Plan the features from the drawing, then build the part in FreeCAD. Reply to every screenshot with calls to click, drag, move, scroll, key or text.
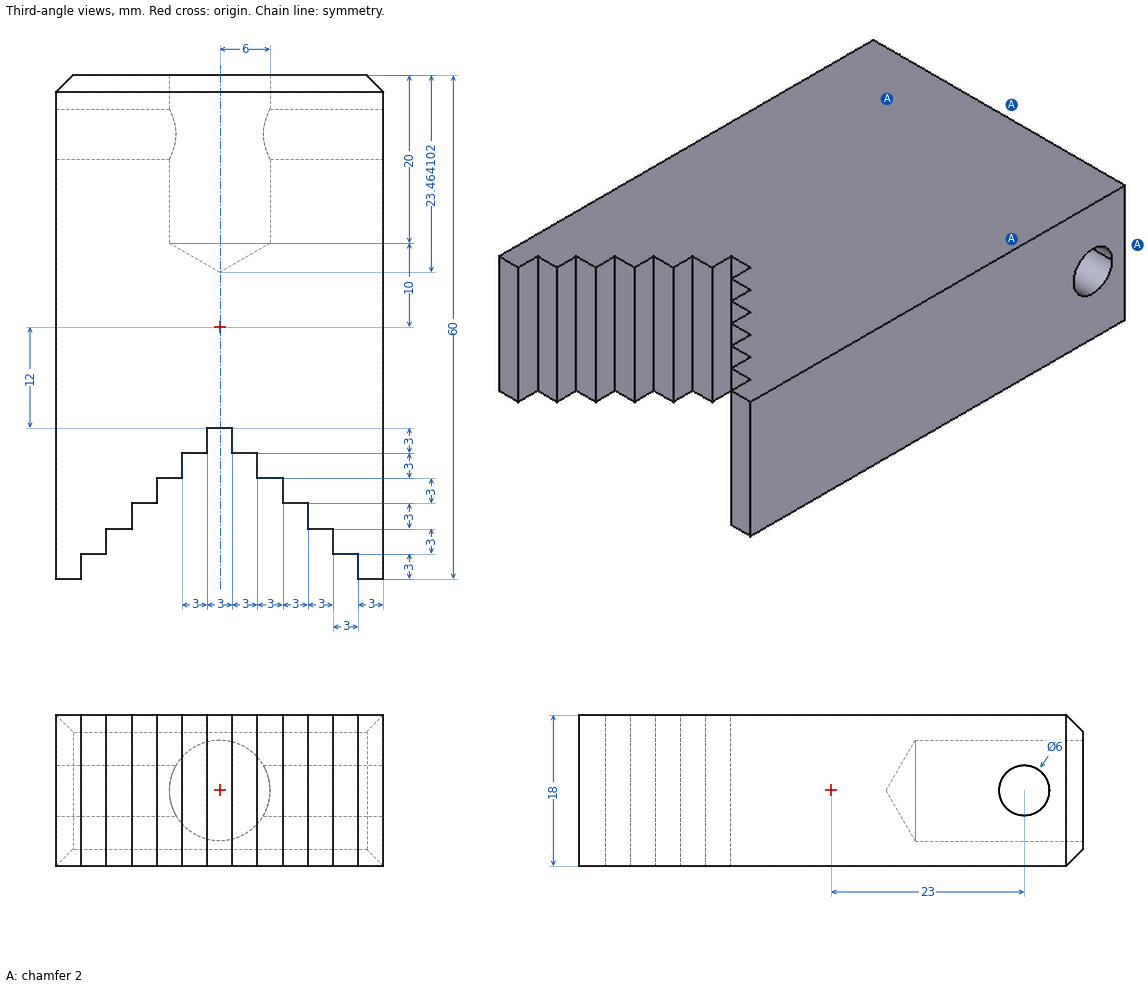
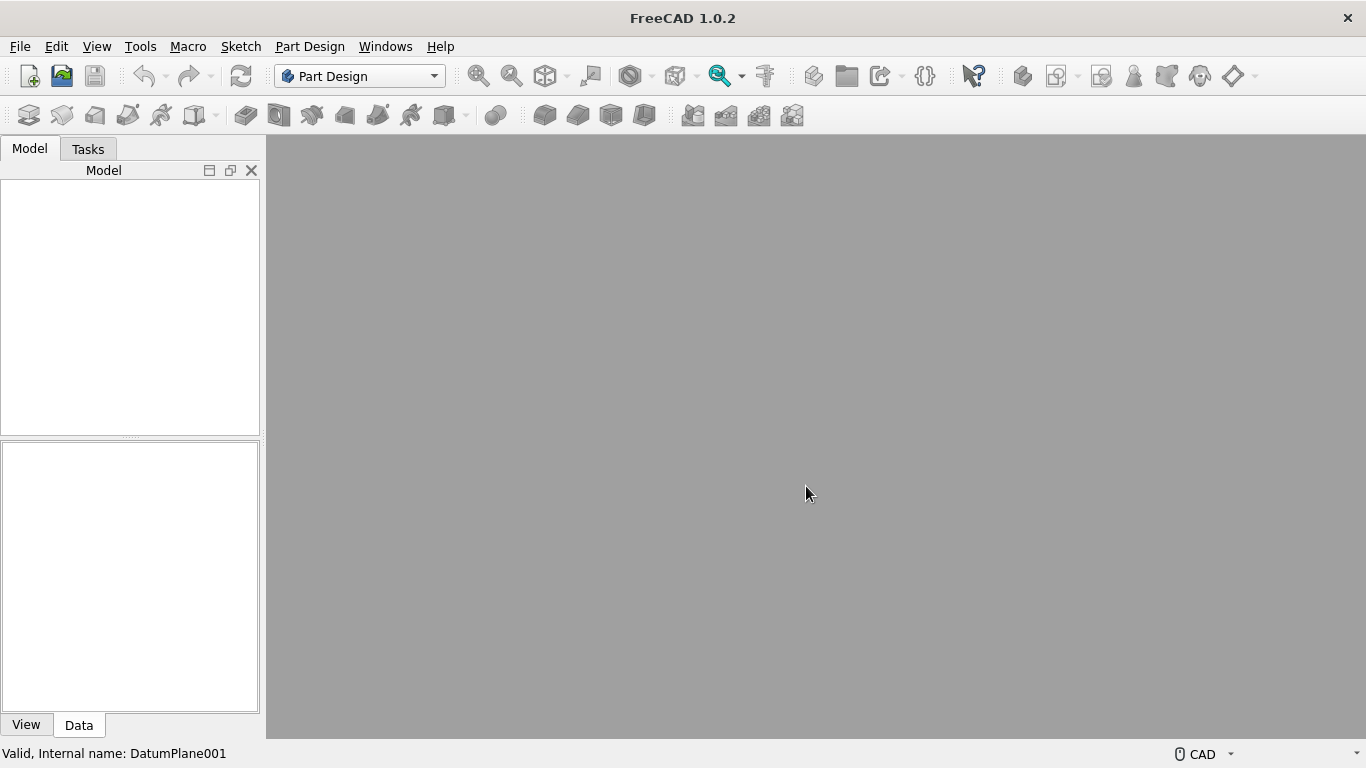
key(ctrl+n)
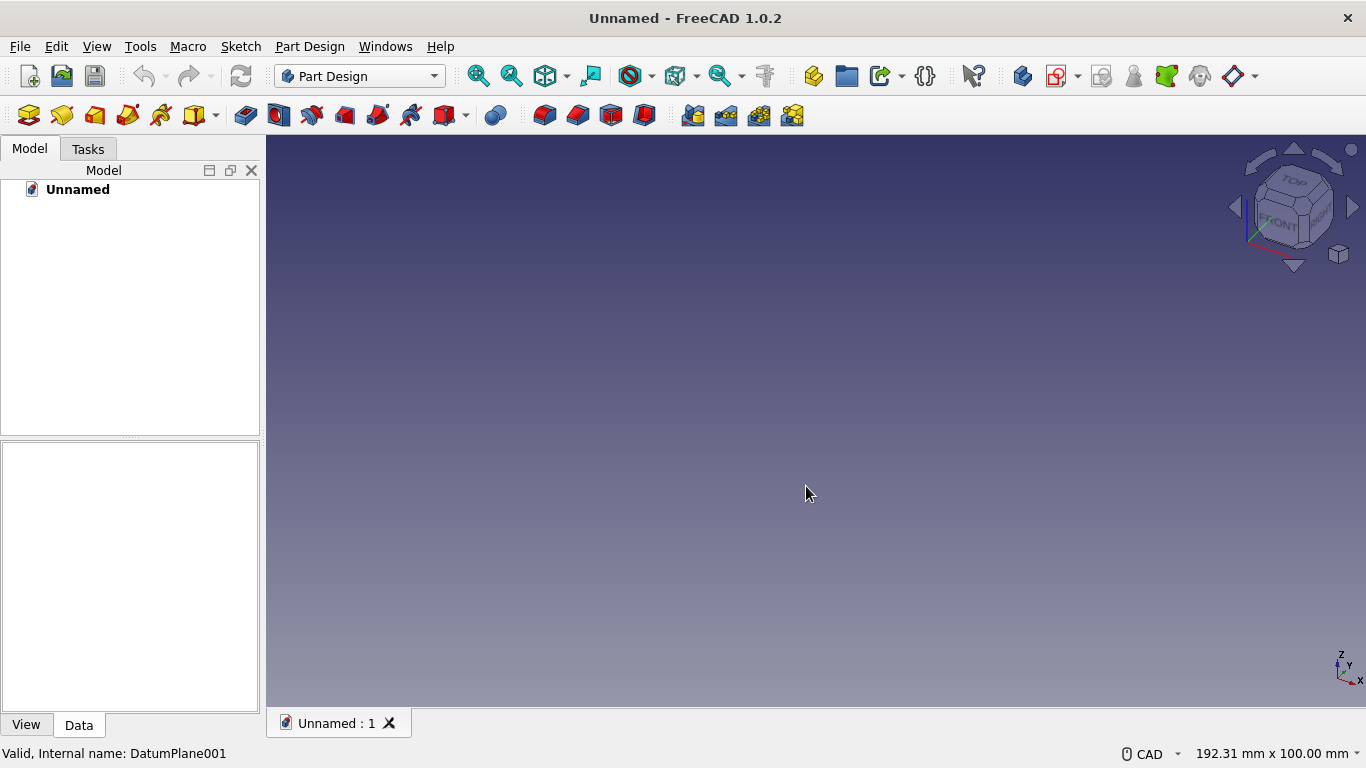
click(1056, 76)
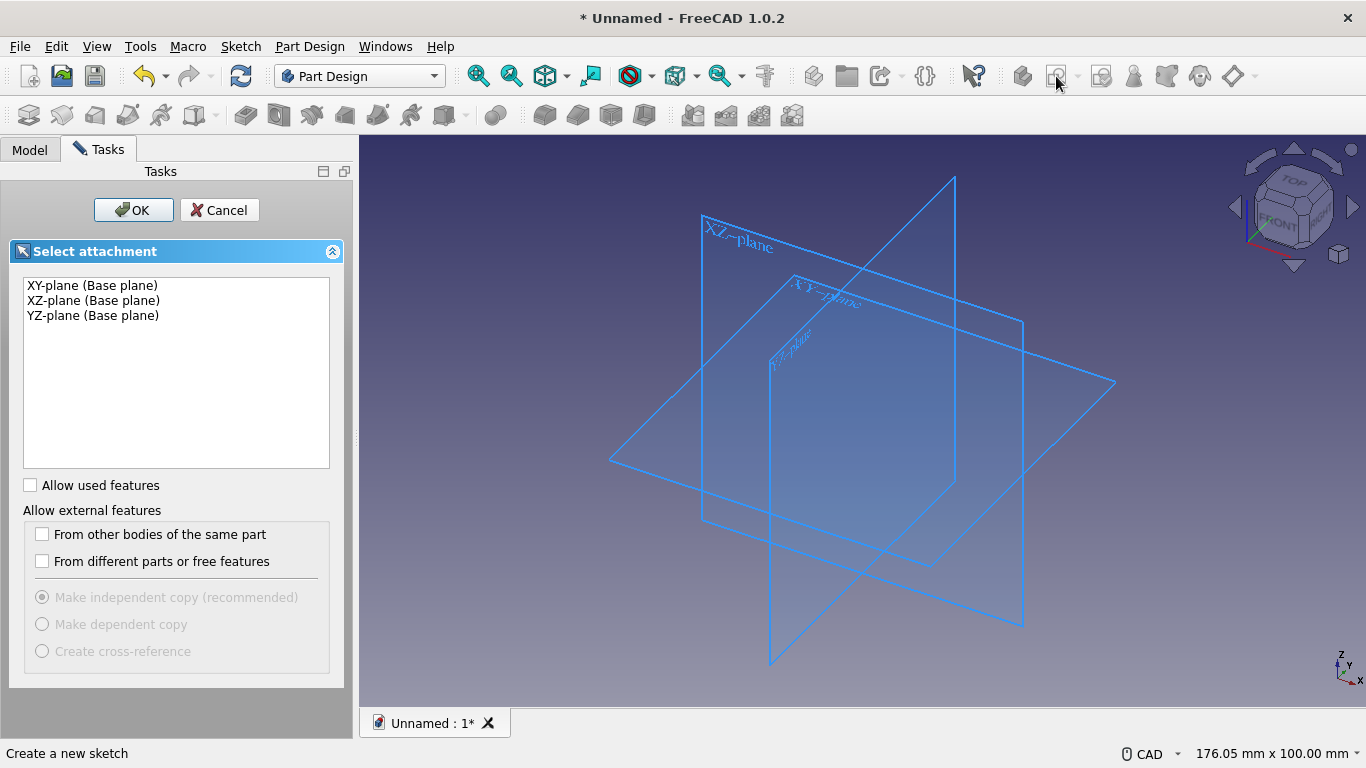
click(84, 286)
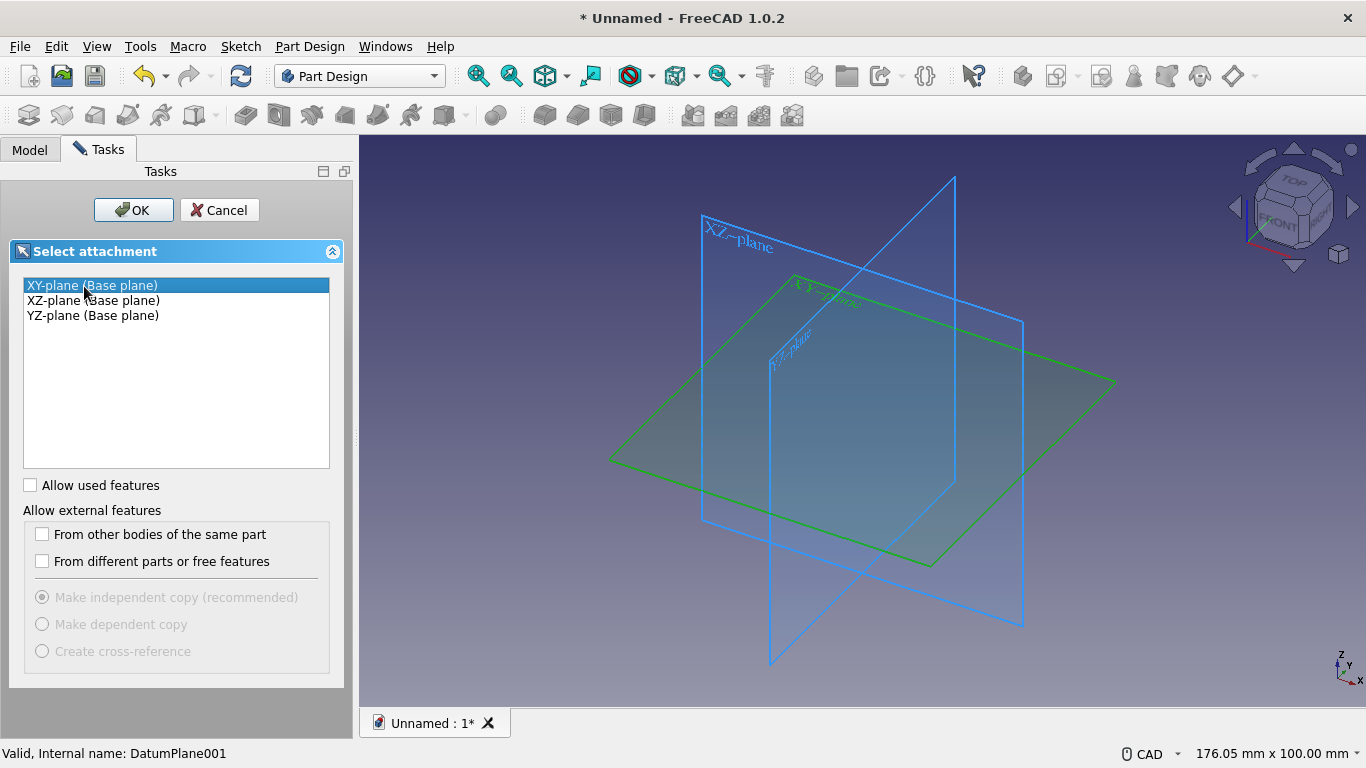
click(134, 210)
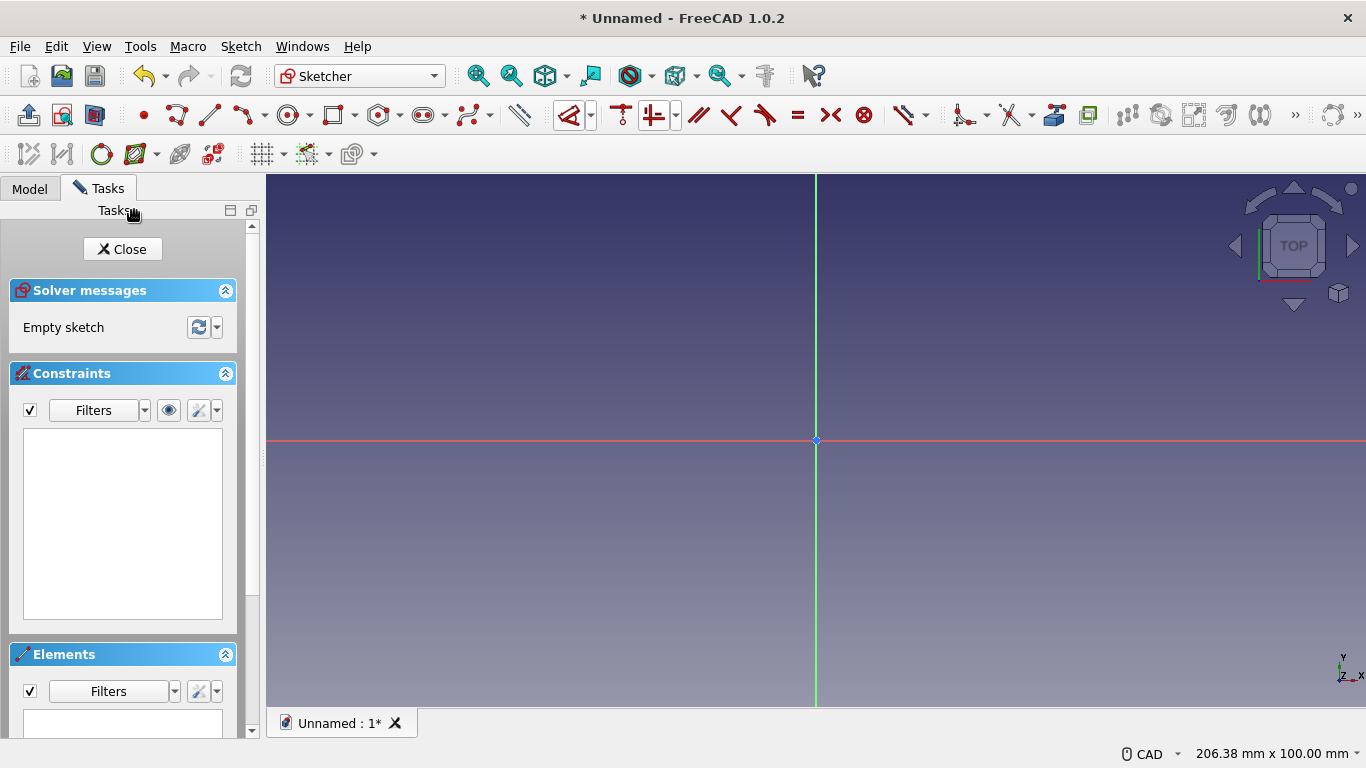
click(177, 116)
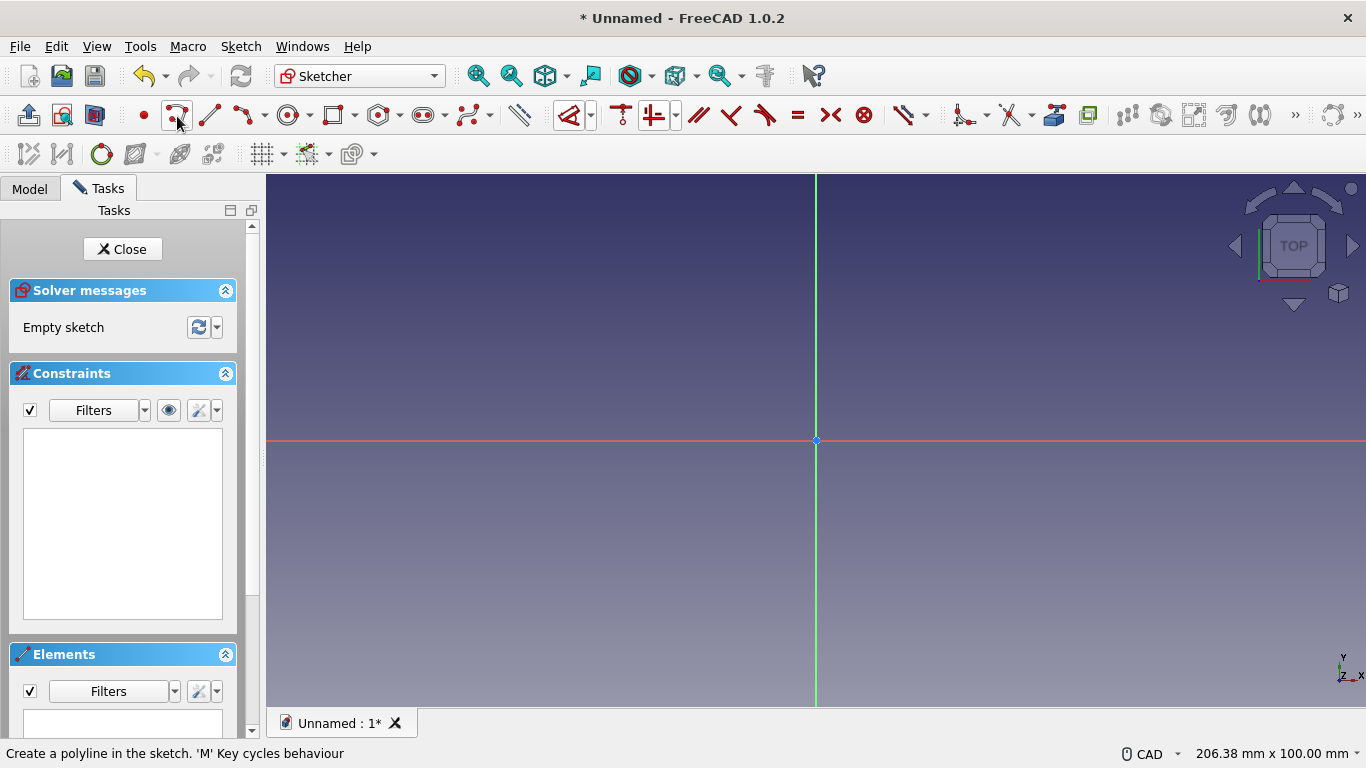
scroll(808, 504, up, 4)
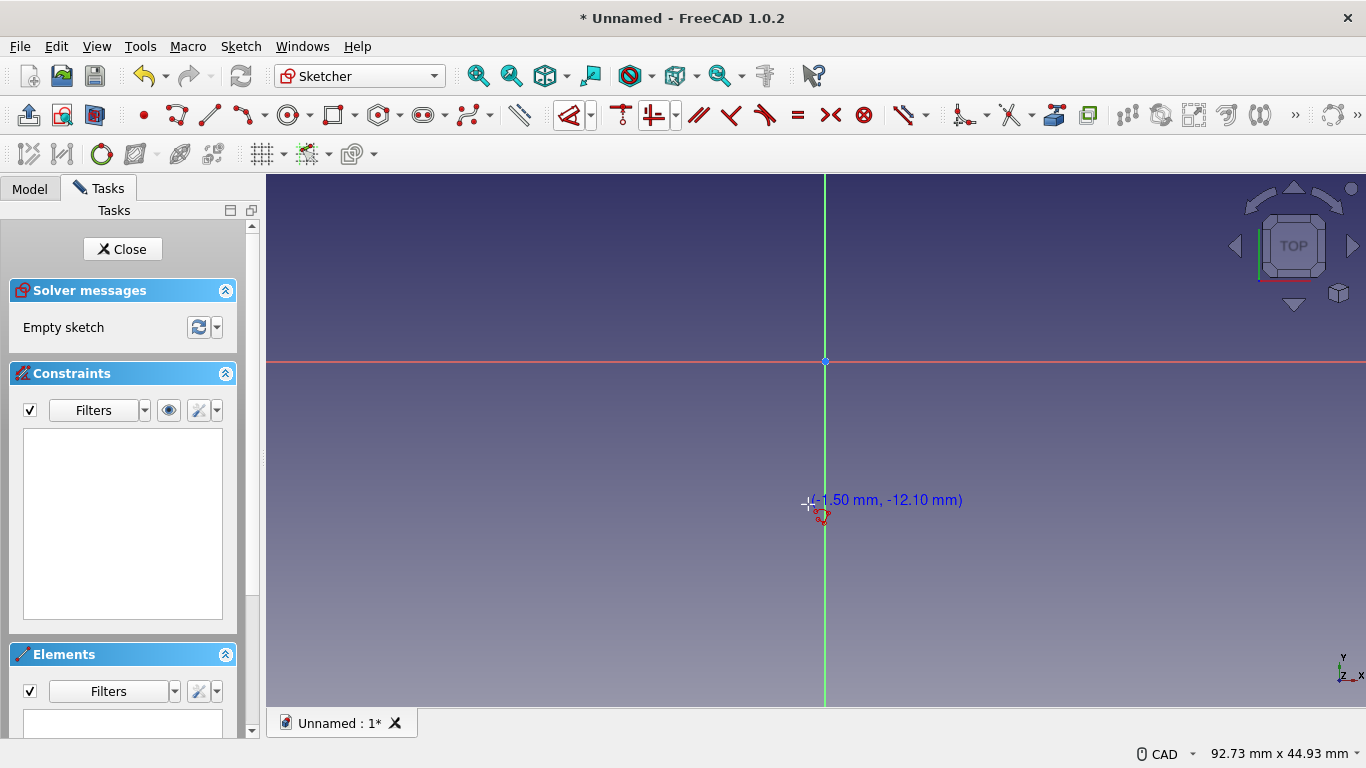
click(807, 504)
click(843, 504)
click(843, 540)
click(879, 540)
click(879, 575)
click(914, 575)
click(914, 611)
click(950, 611)
click(950, 647)
click(985, 647)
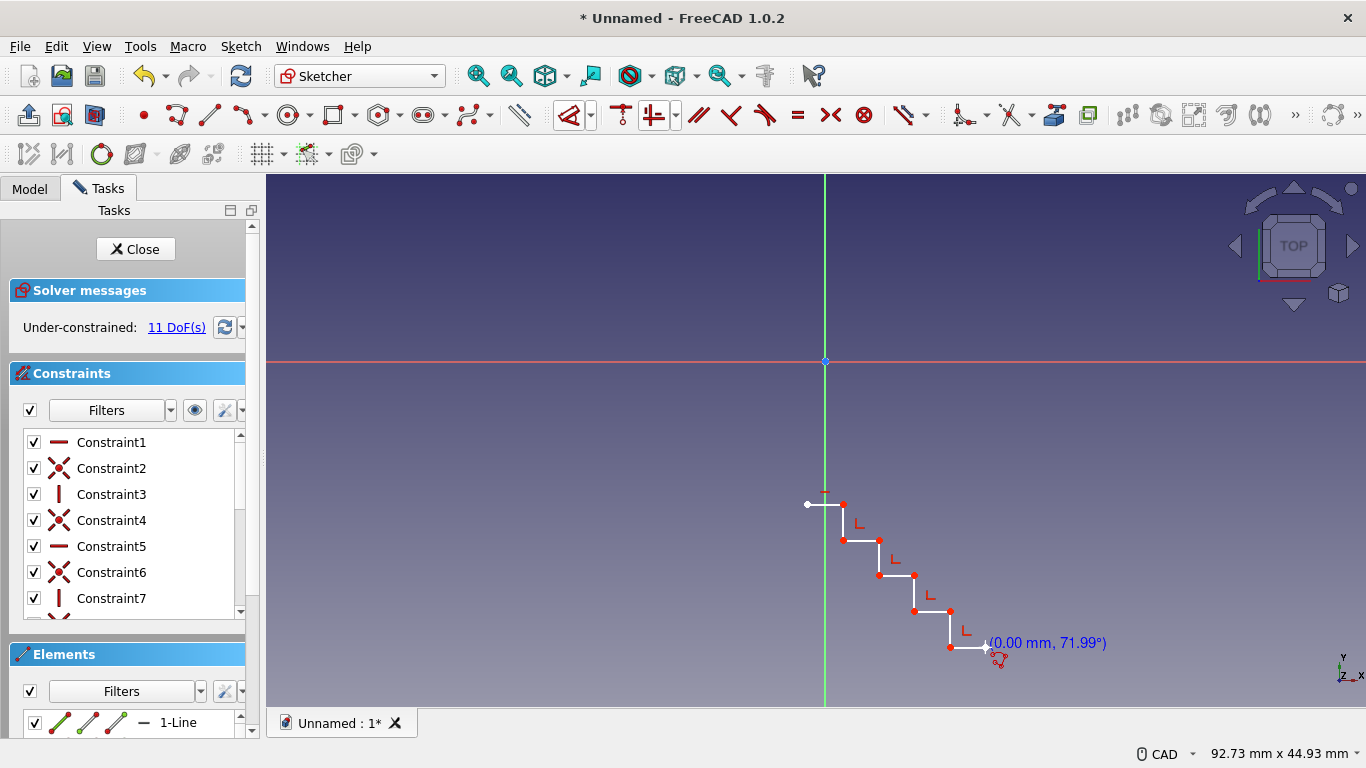
scroll(684, 505, down, 4)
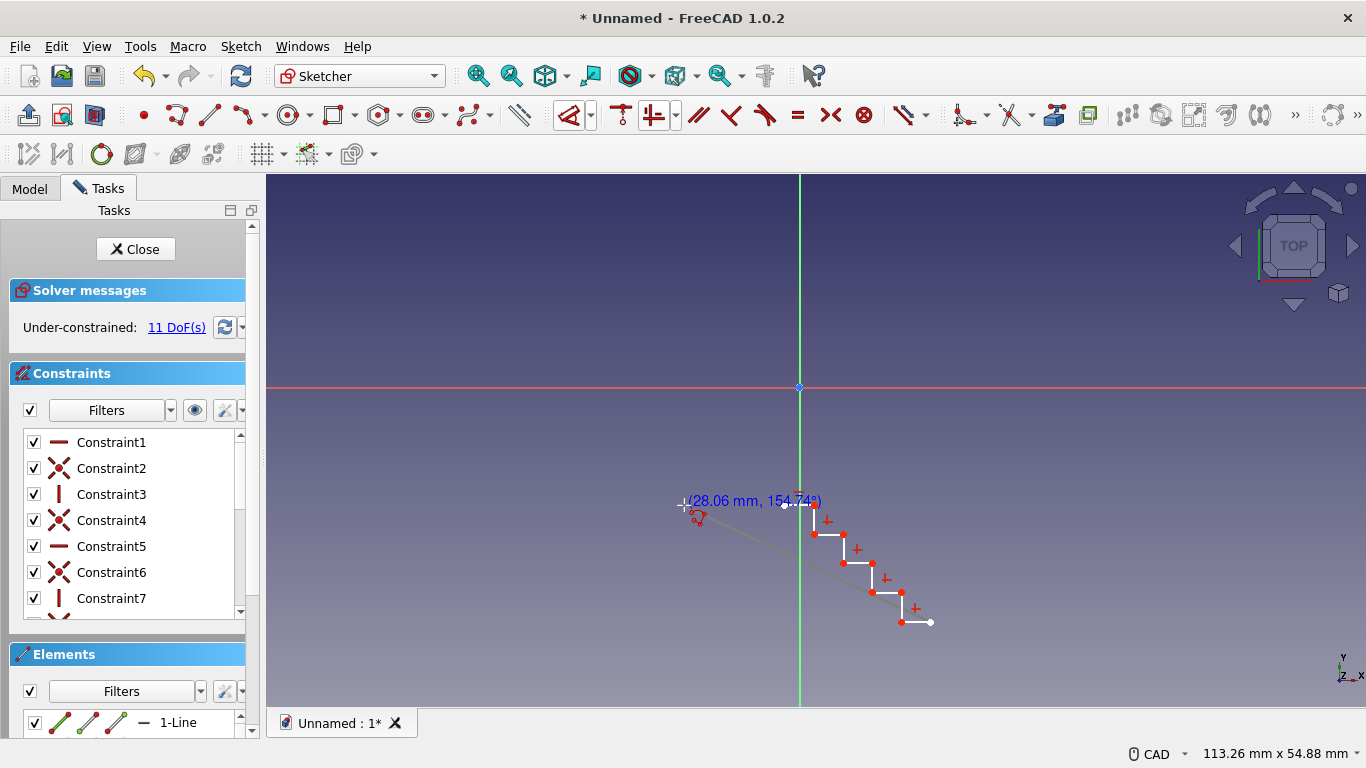
click(819, 585)
click(836, 585)
click(836, 601)
click(852, 601)
click(852, 281)
click(644, 281)
click(644, 601)
click(660, 601)
click(660, 585)
click(676, 585)
click(676, 569)
click(692, 569)
click(692, 553)
click(708, 553)
click(708, 537)
click(724, 537)
click(724, 521)